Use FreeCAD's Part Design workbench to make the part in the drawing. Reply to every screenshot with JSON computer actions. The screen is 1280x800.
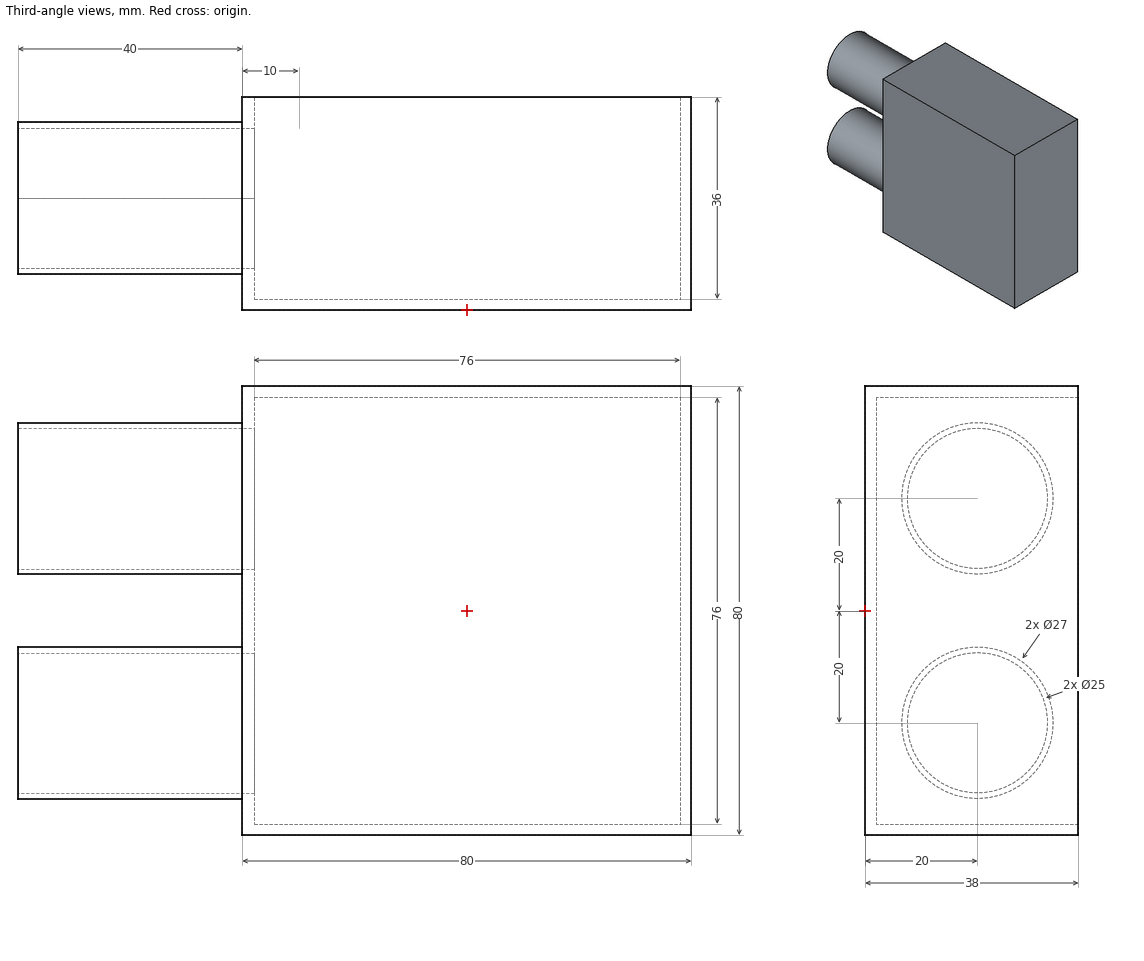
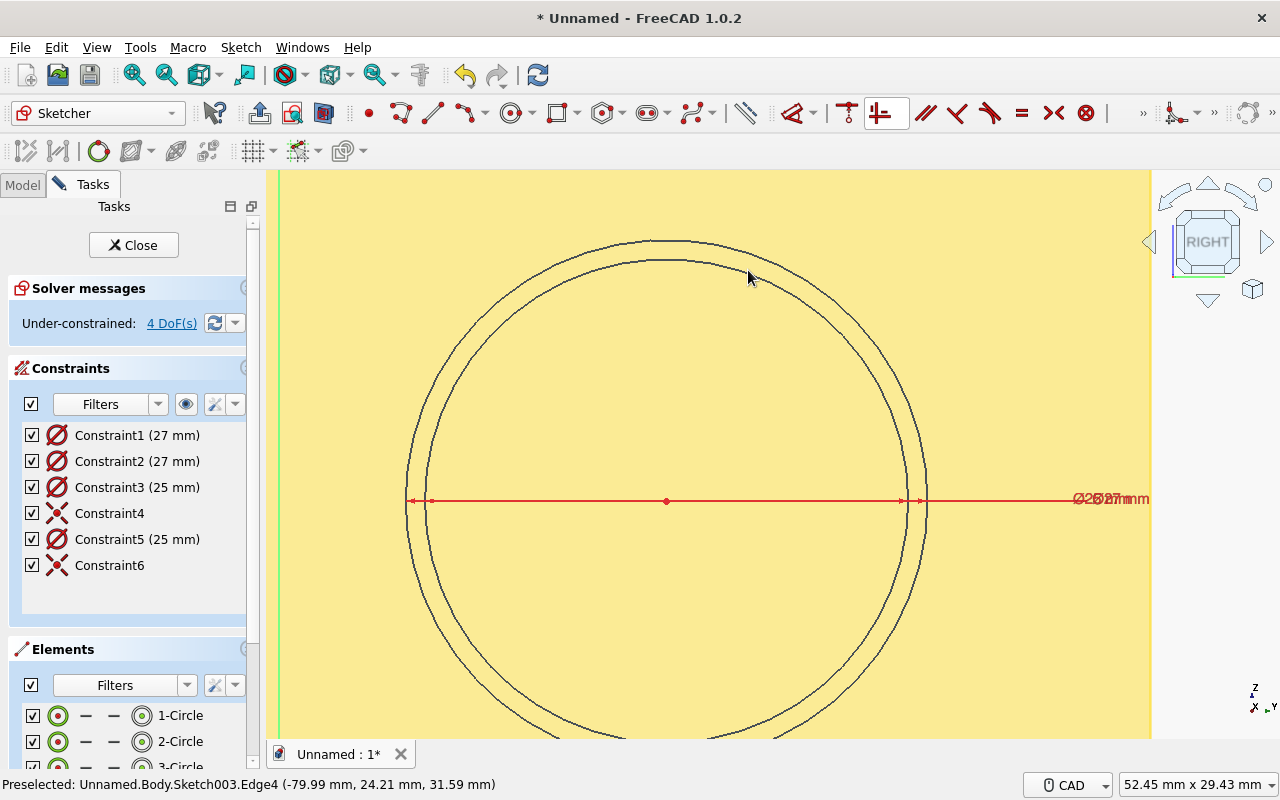
{"action": "scroll", "coordinate": [748, 269], "scroll_direction": "down", "scroll_amount": 6}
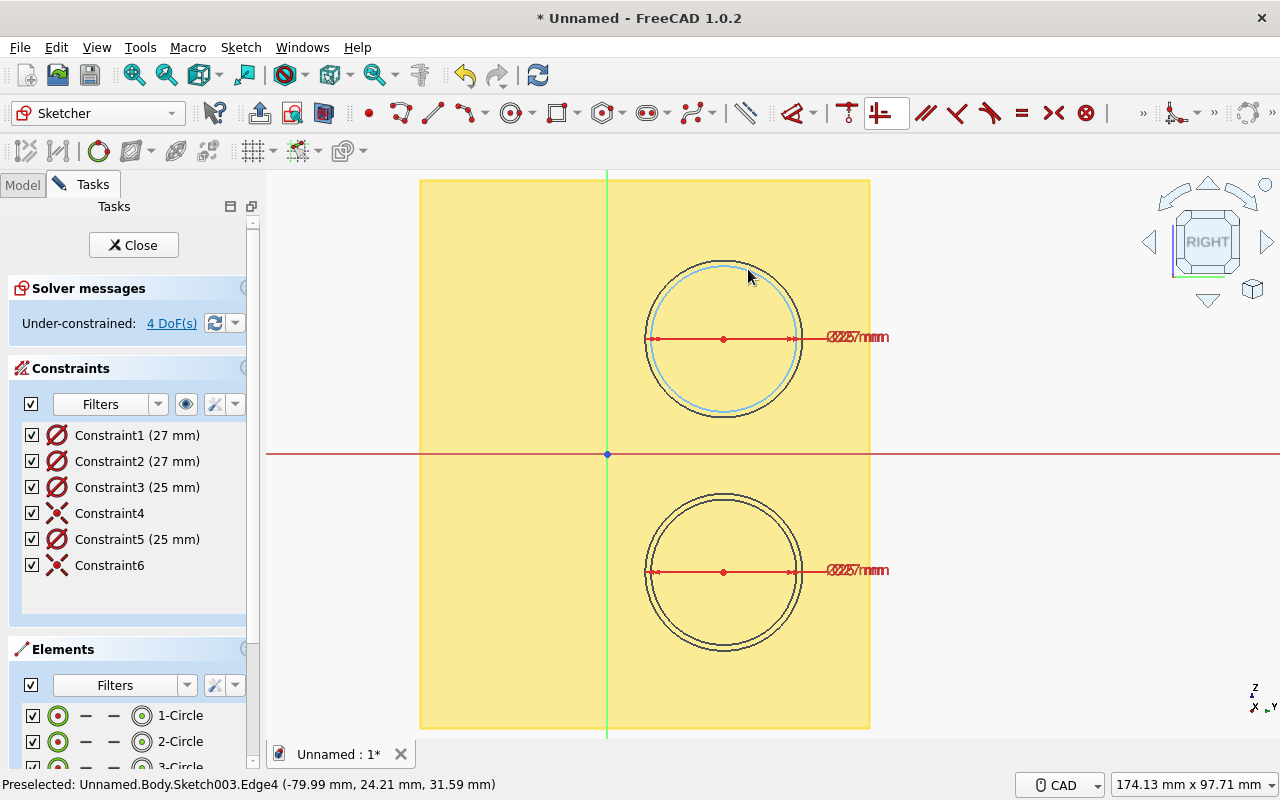
{"action": "left_click", "coordinate": [724, 572]}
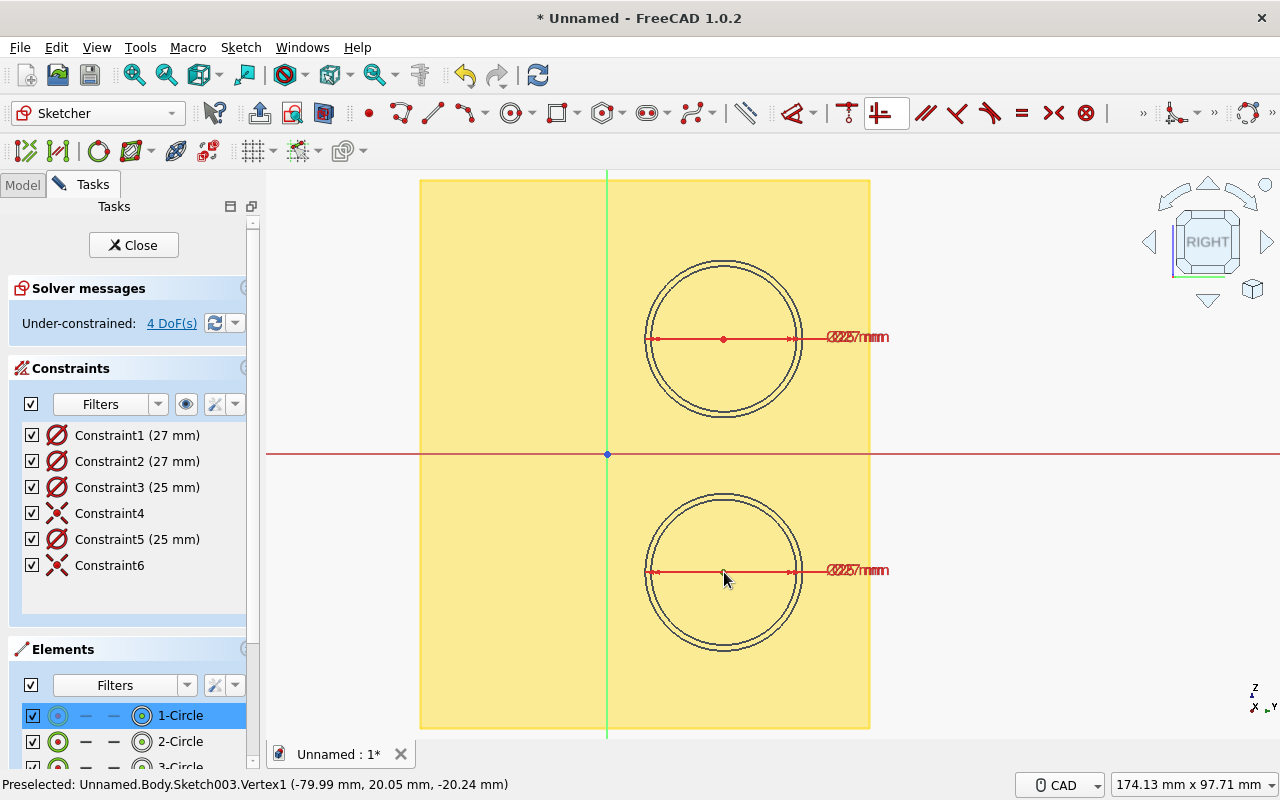
{"action": "left_click", "coordinate": [724, 339]}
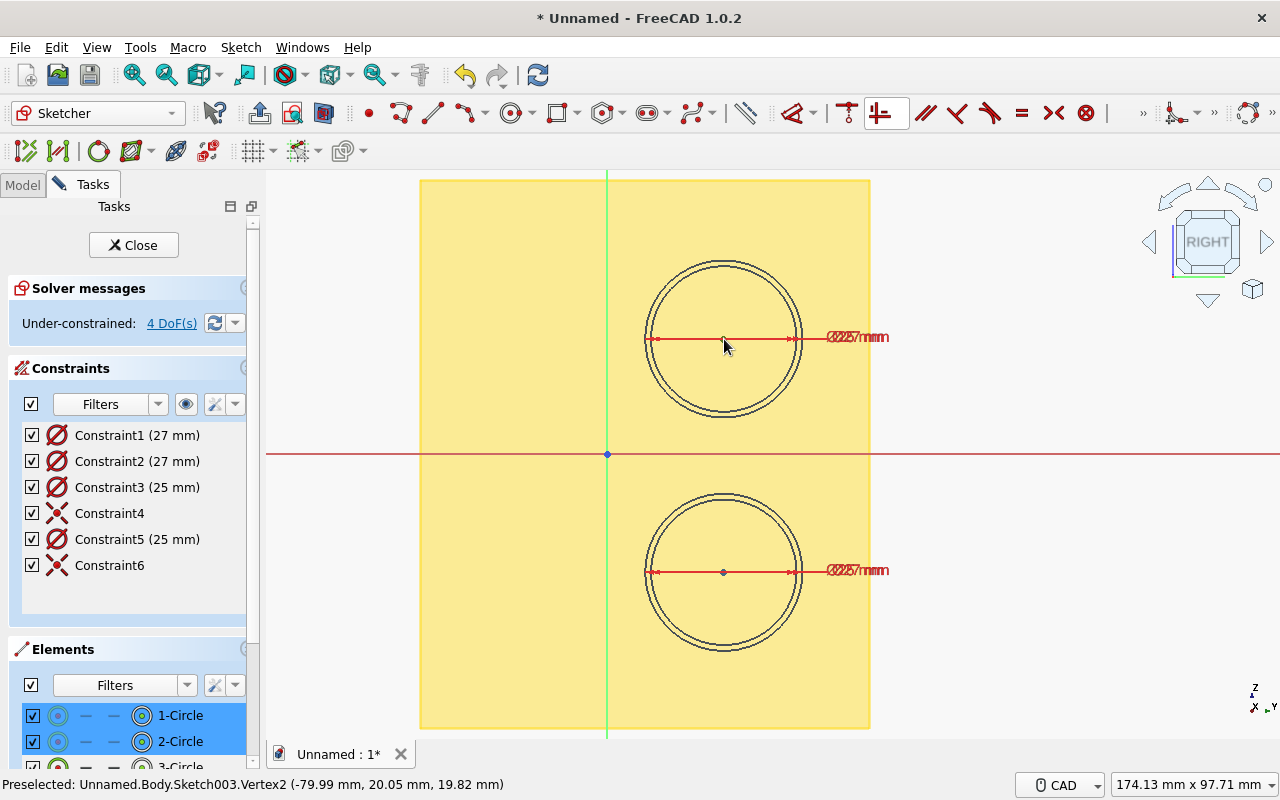
{"action": "key", "text": "v"}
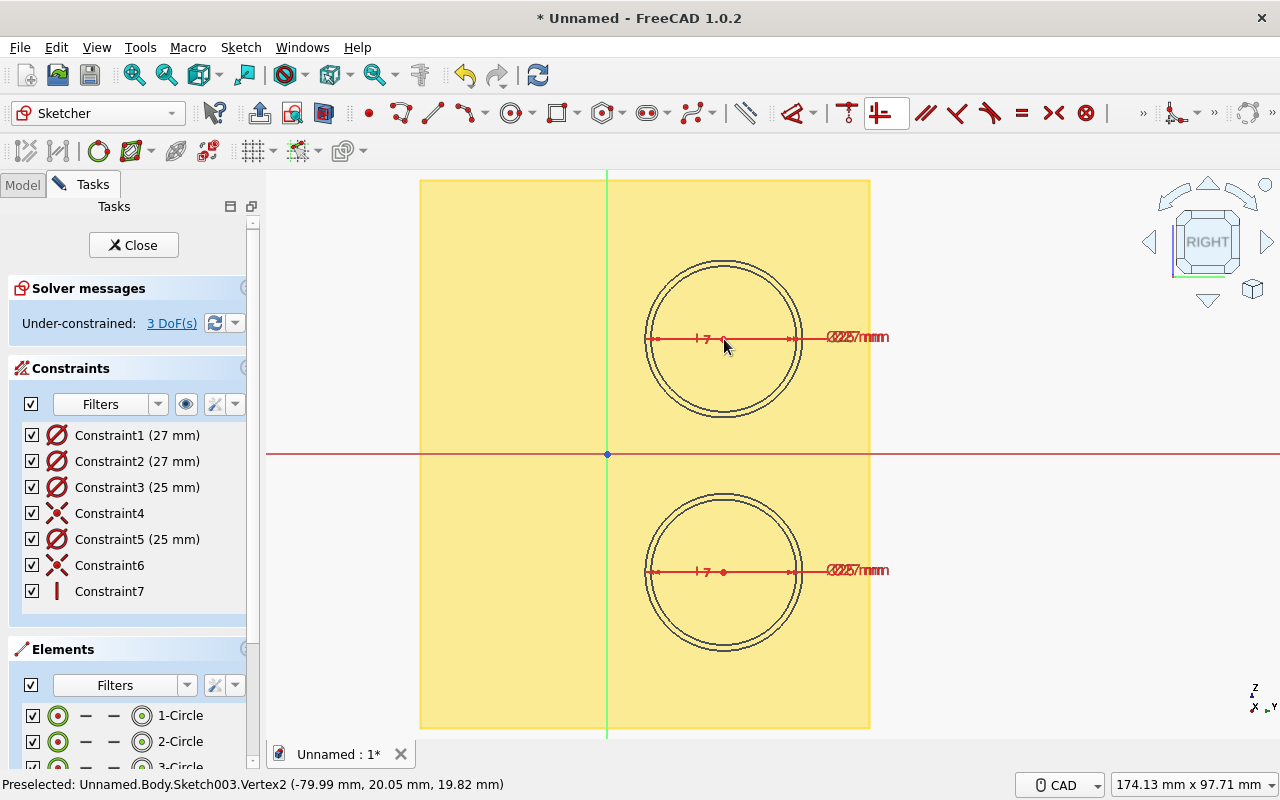
{"action": "left_click", "coordinate": [792, 114]}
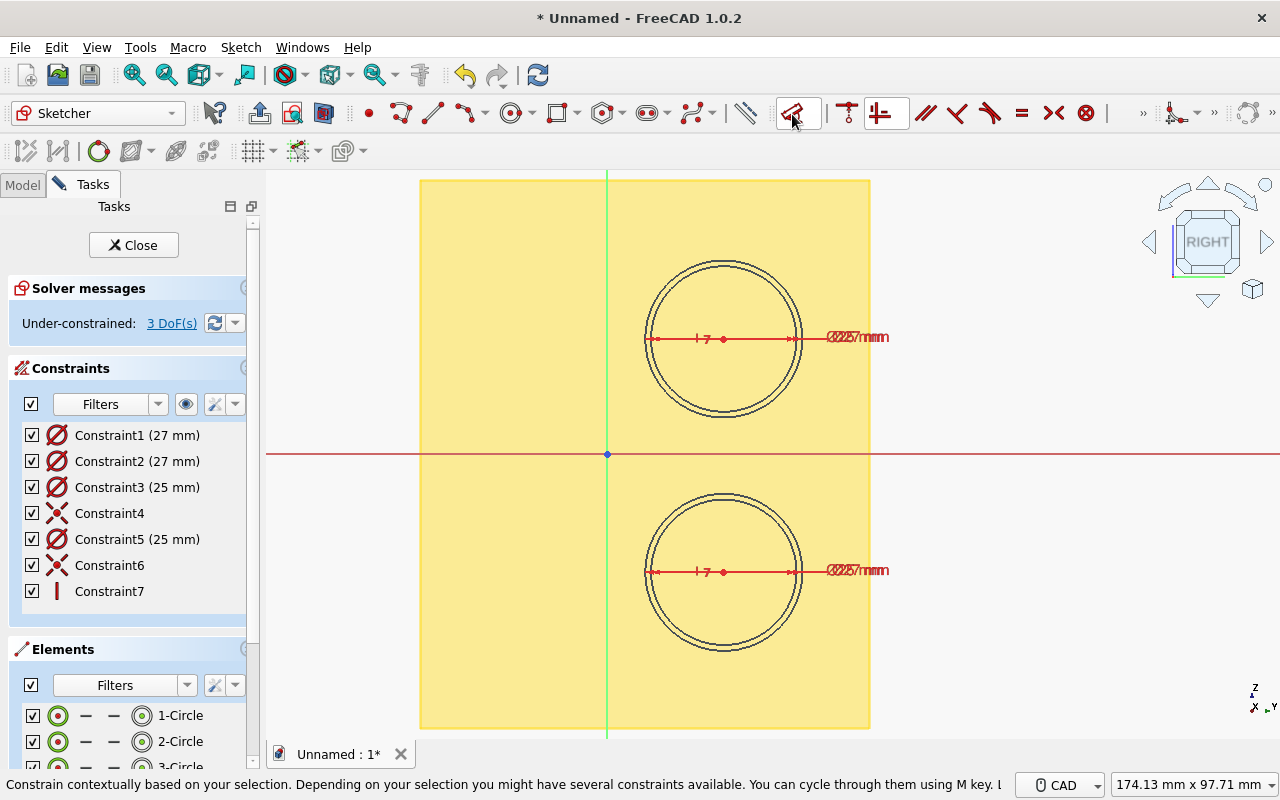
{"action": "left_click", "coordinate": [724, 572]}
{"action": "left_click", "coordinate": [639, 606]}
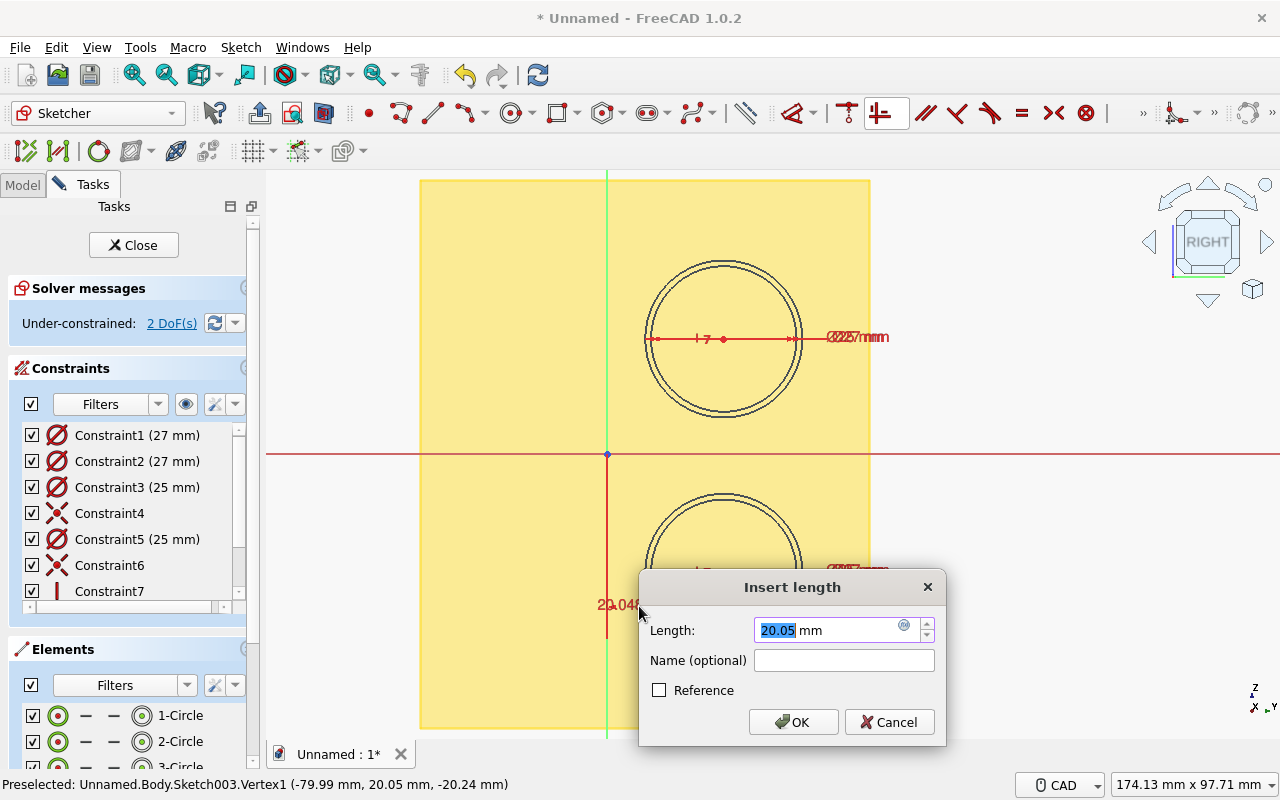
{"action": "type", "text": "20"}
{"action": "key", "text": "Return"}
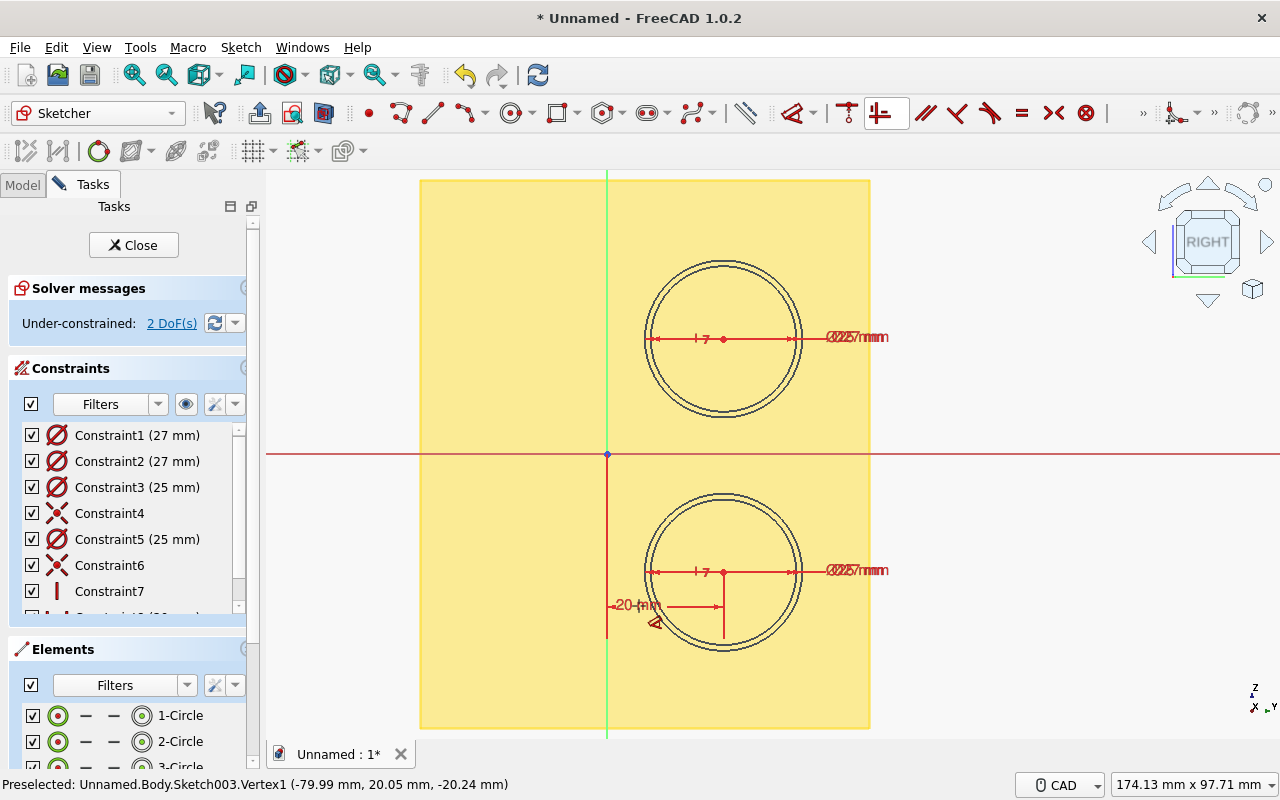
{"action": "left_click", "coordinate": [724, 572]}
{"action": "left_click", "coordinate": [573, 513]}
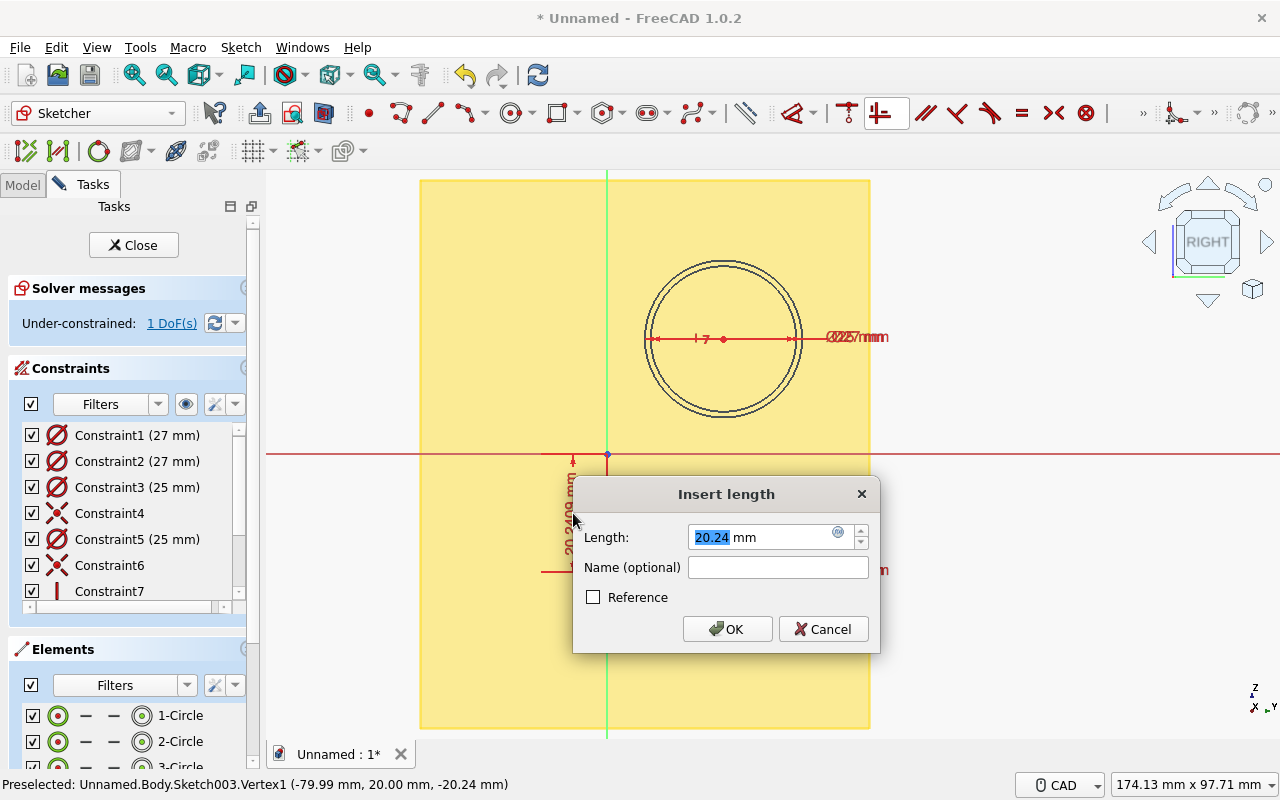
{"action": "type", "text": "20"}
{"action": "key", "text": "Return"}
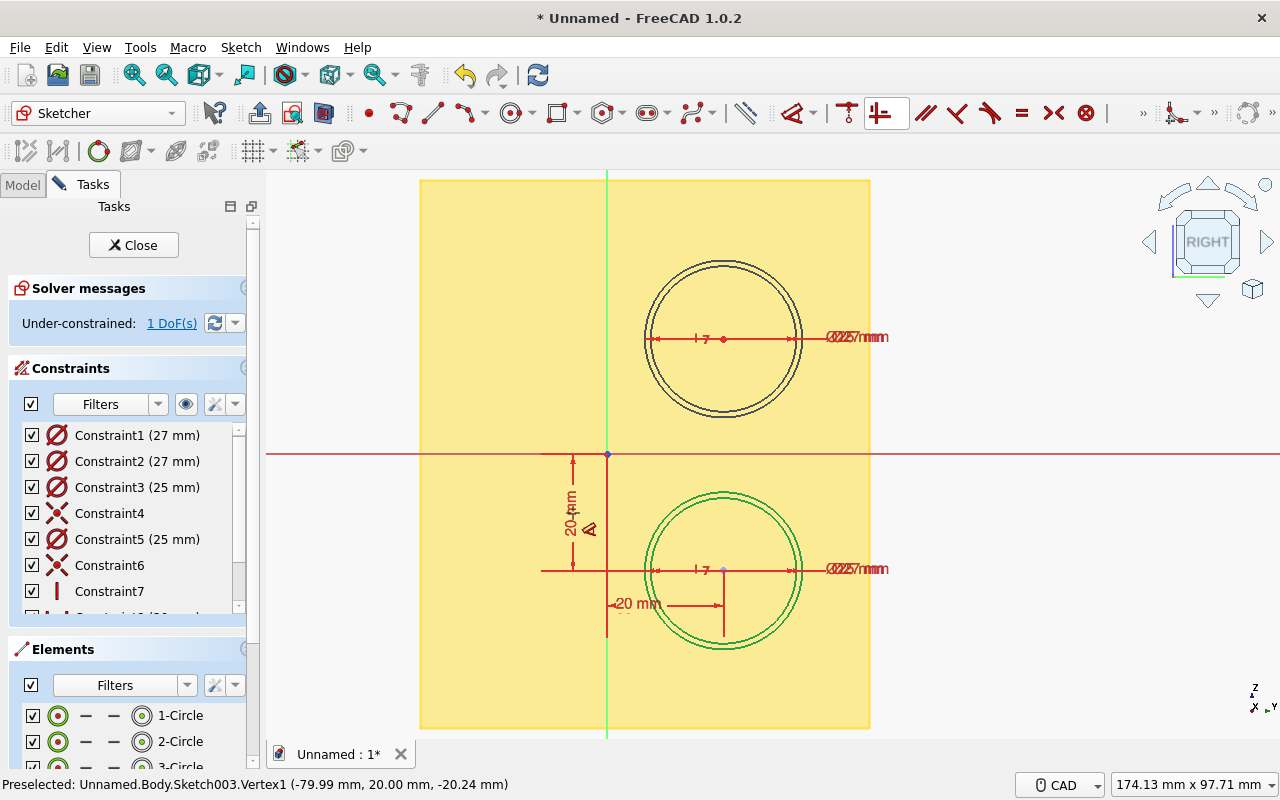
{"action": "left_click", "coordinate": [724, 339]}
{"action": "left_click", "coordinate": [573, 397]}